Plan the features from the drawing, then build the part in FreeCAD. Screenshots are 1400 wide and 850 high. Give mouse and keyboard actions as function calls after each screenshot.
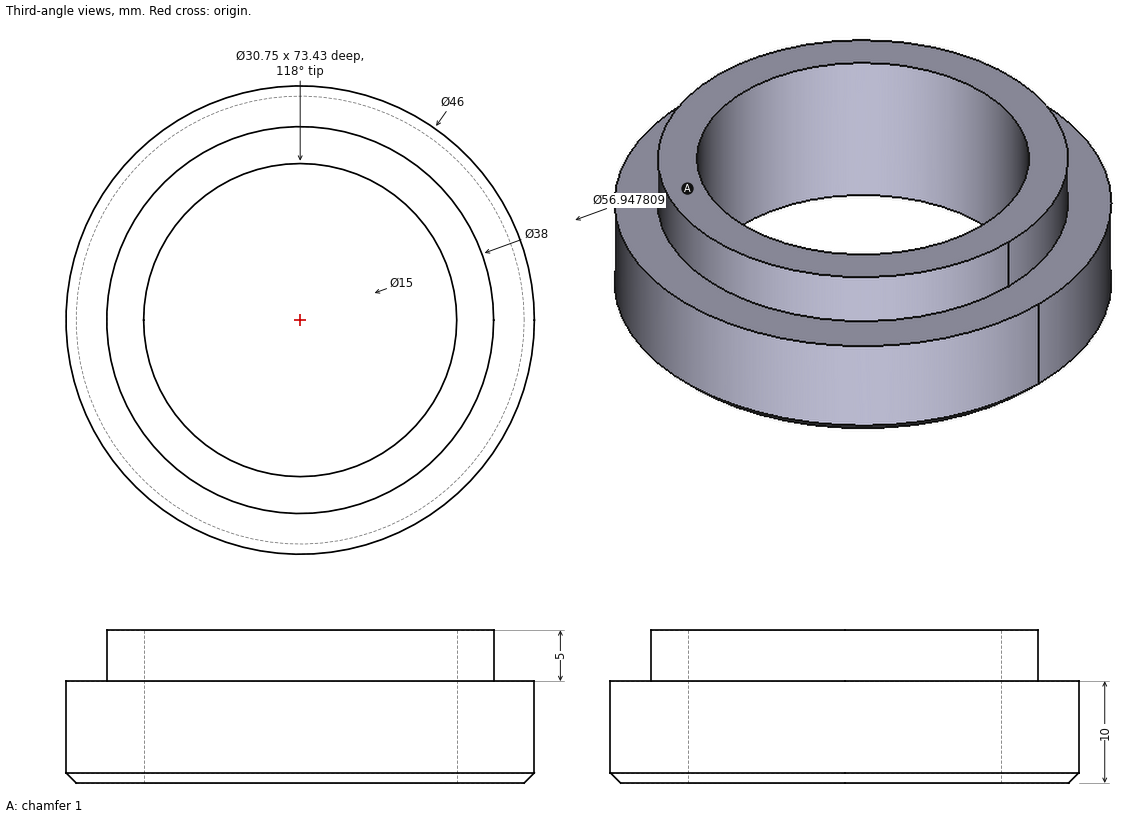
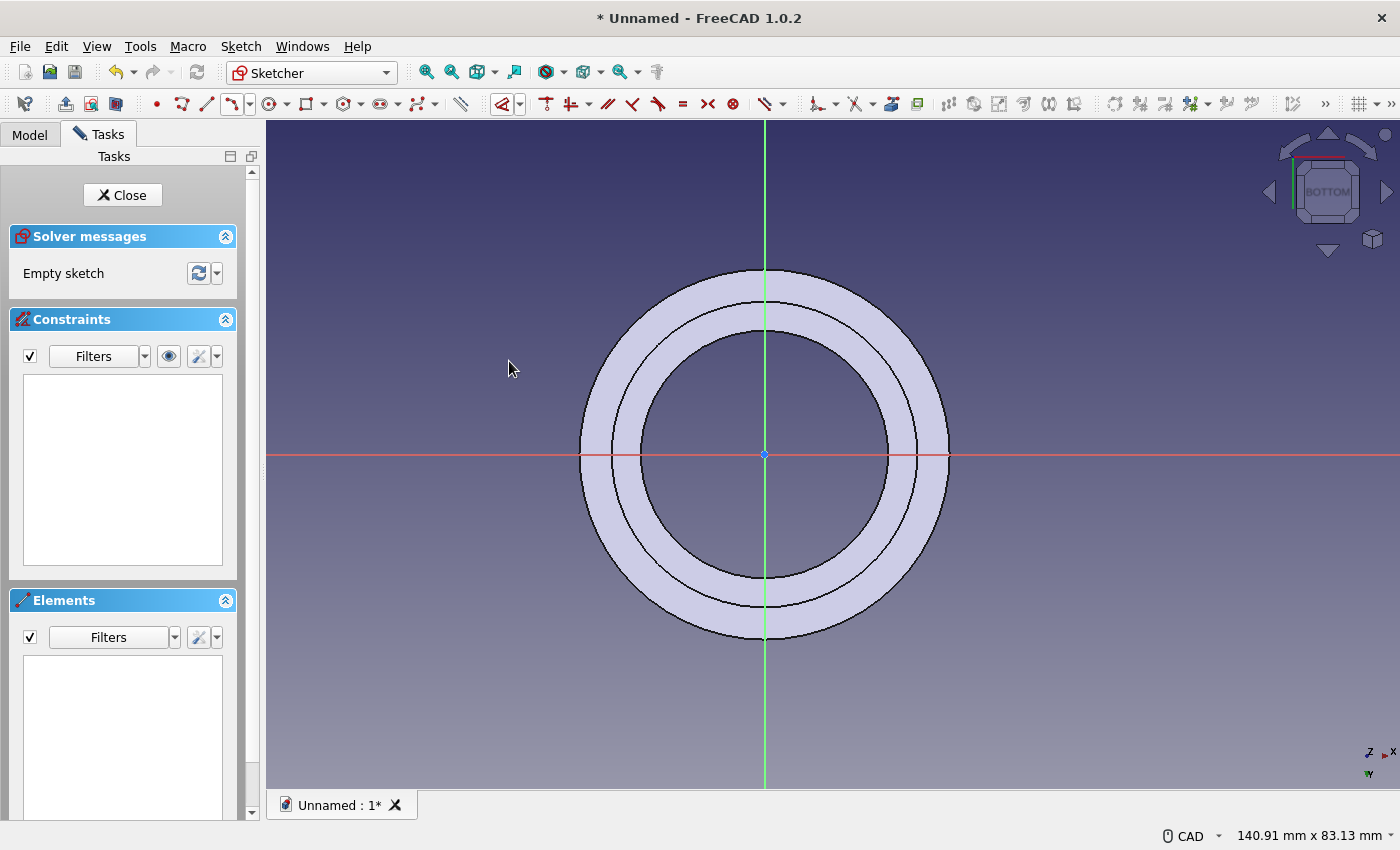
click(268, 104)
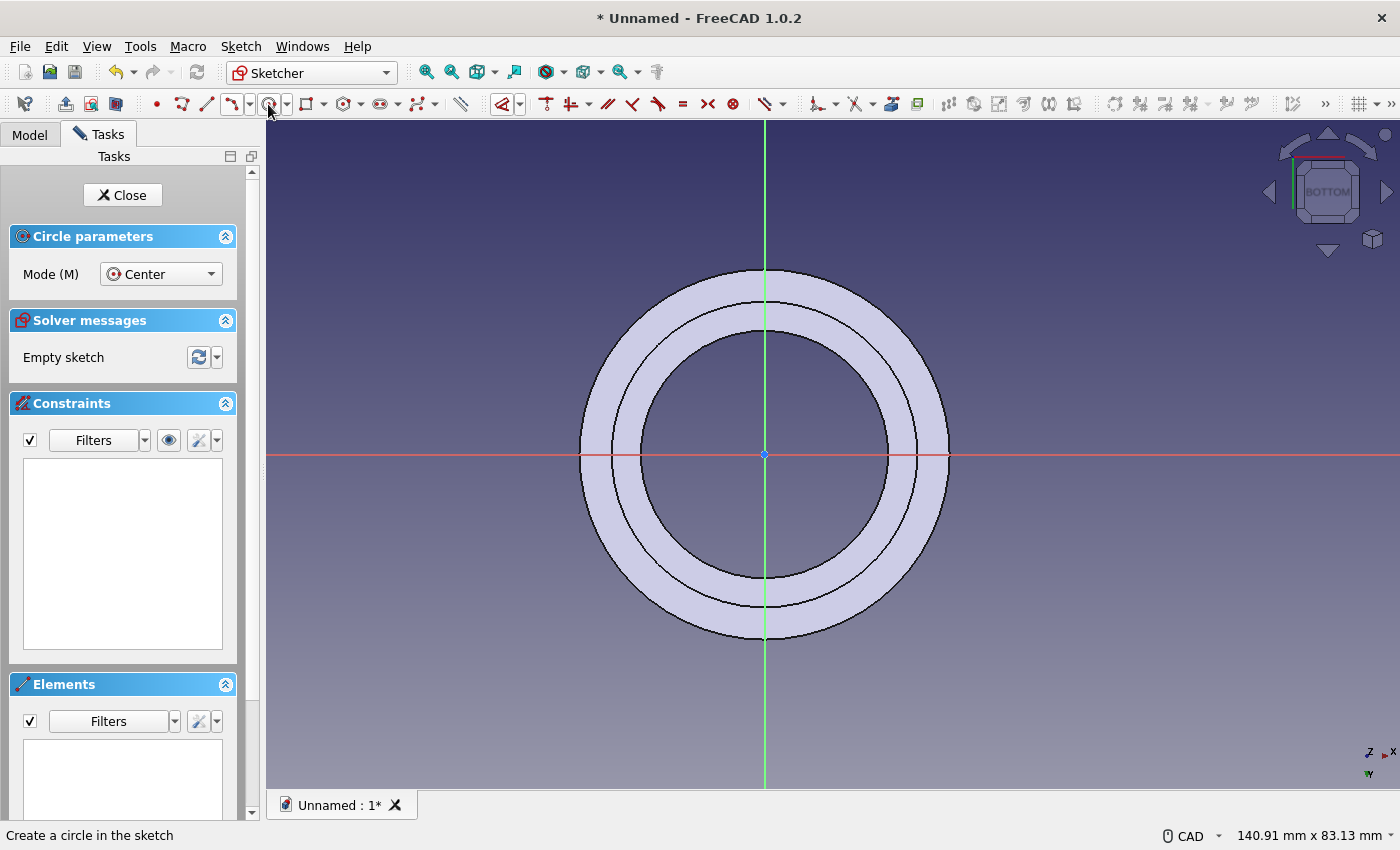
click(765, 455)
move(927, 292)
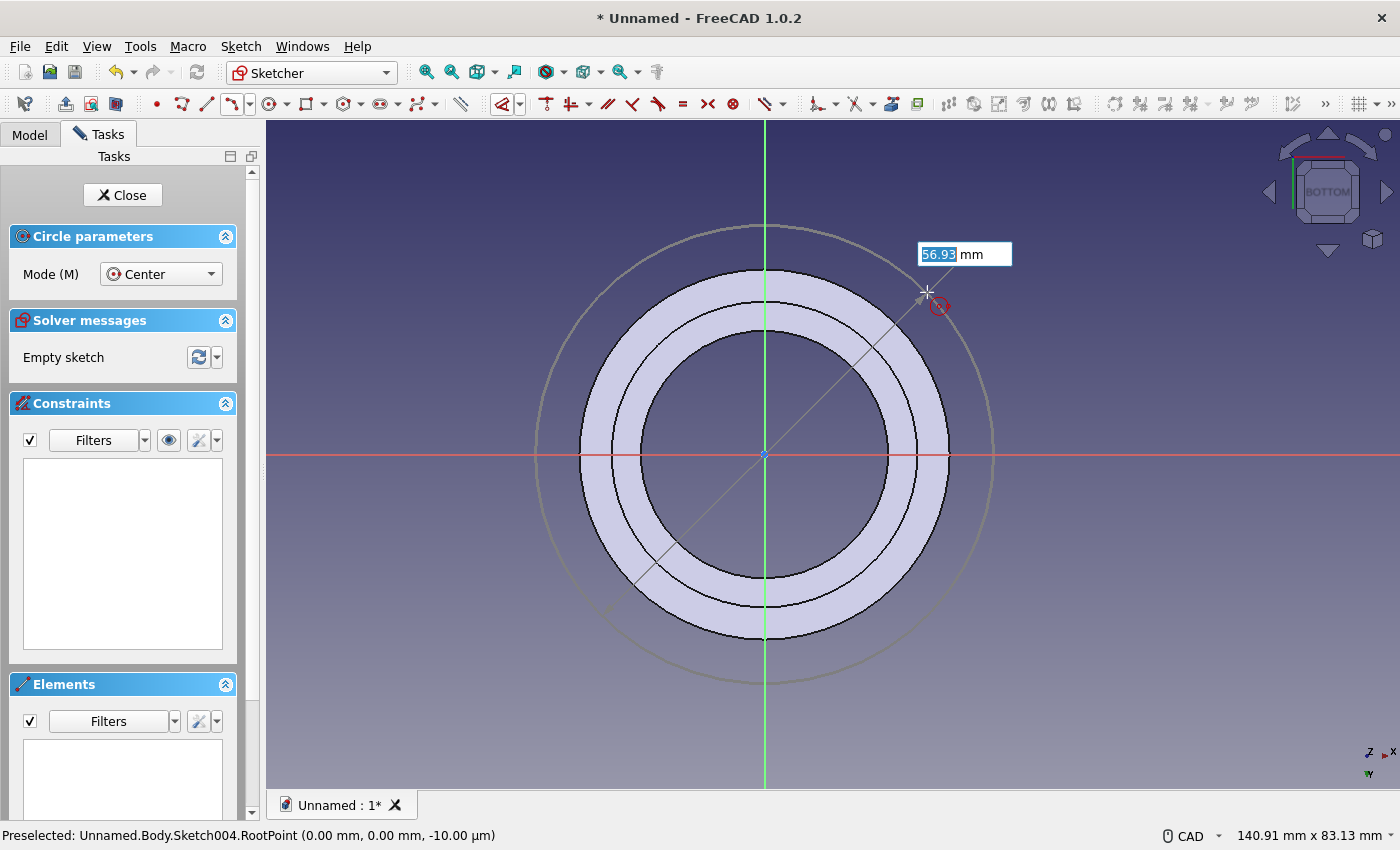
text(56.947809)
key(Return)
key(Escape)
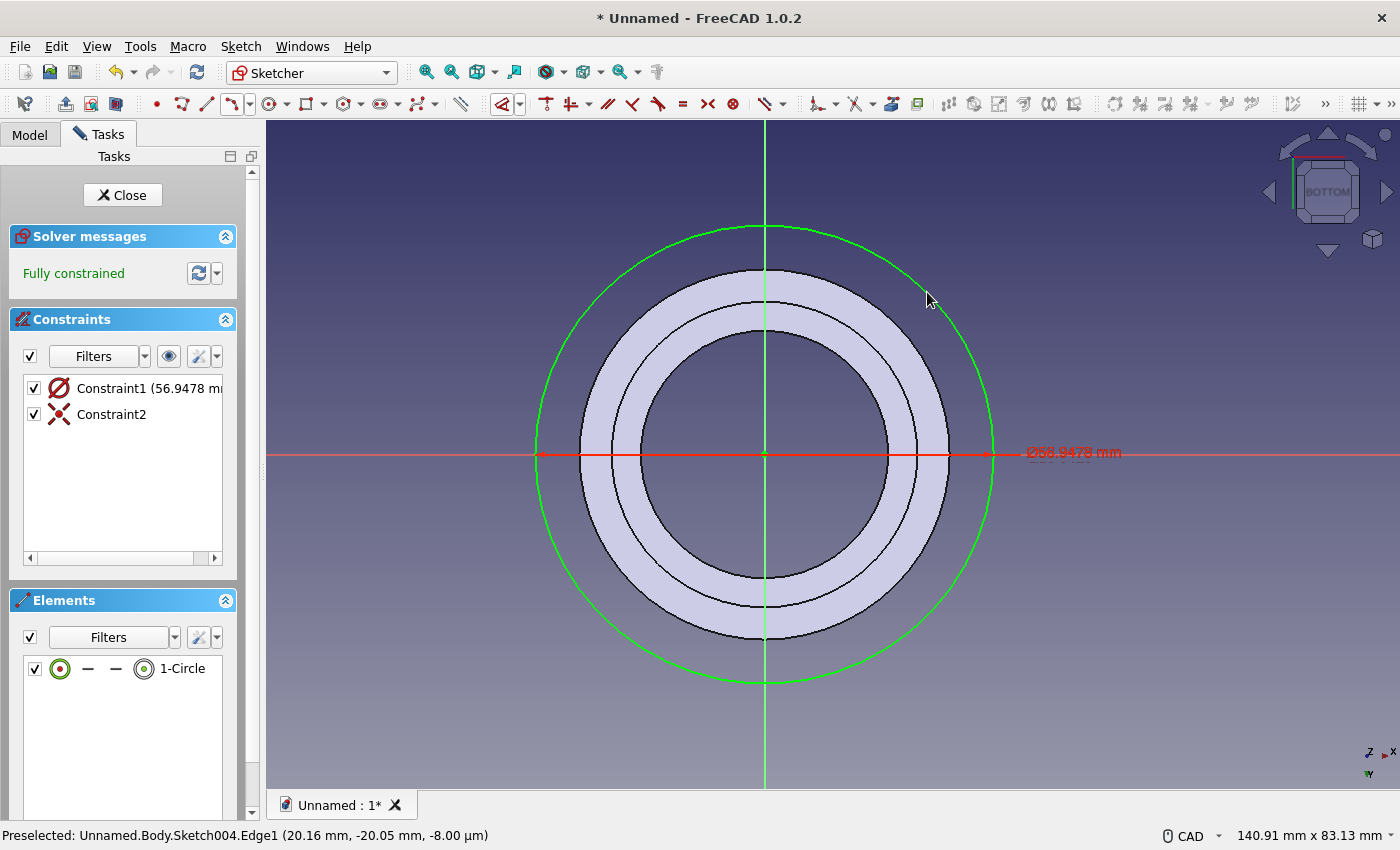
click(123, 195)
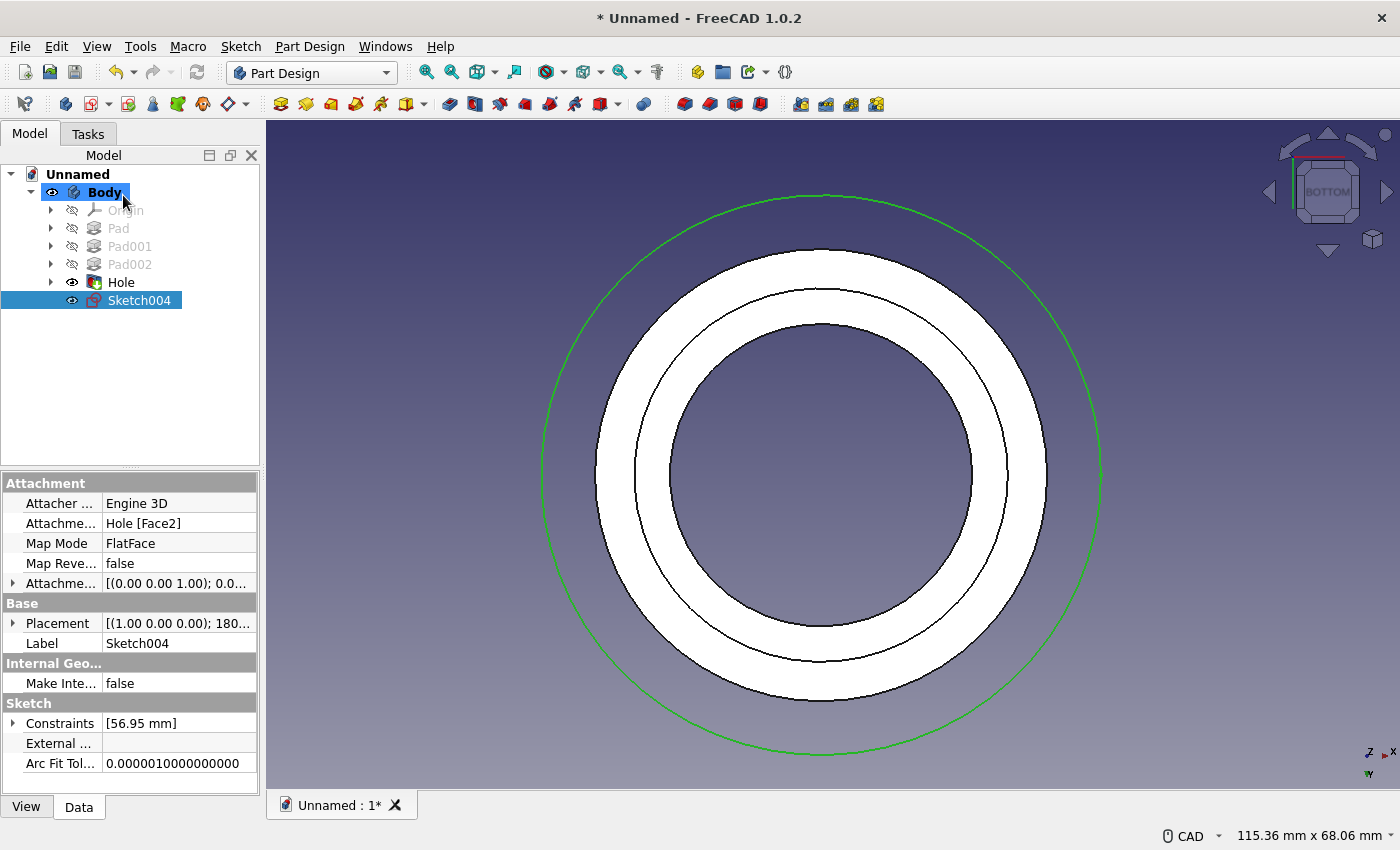
click(450, 104)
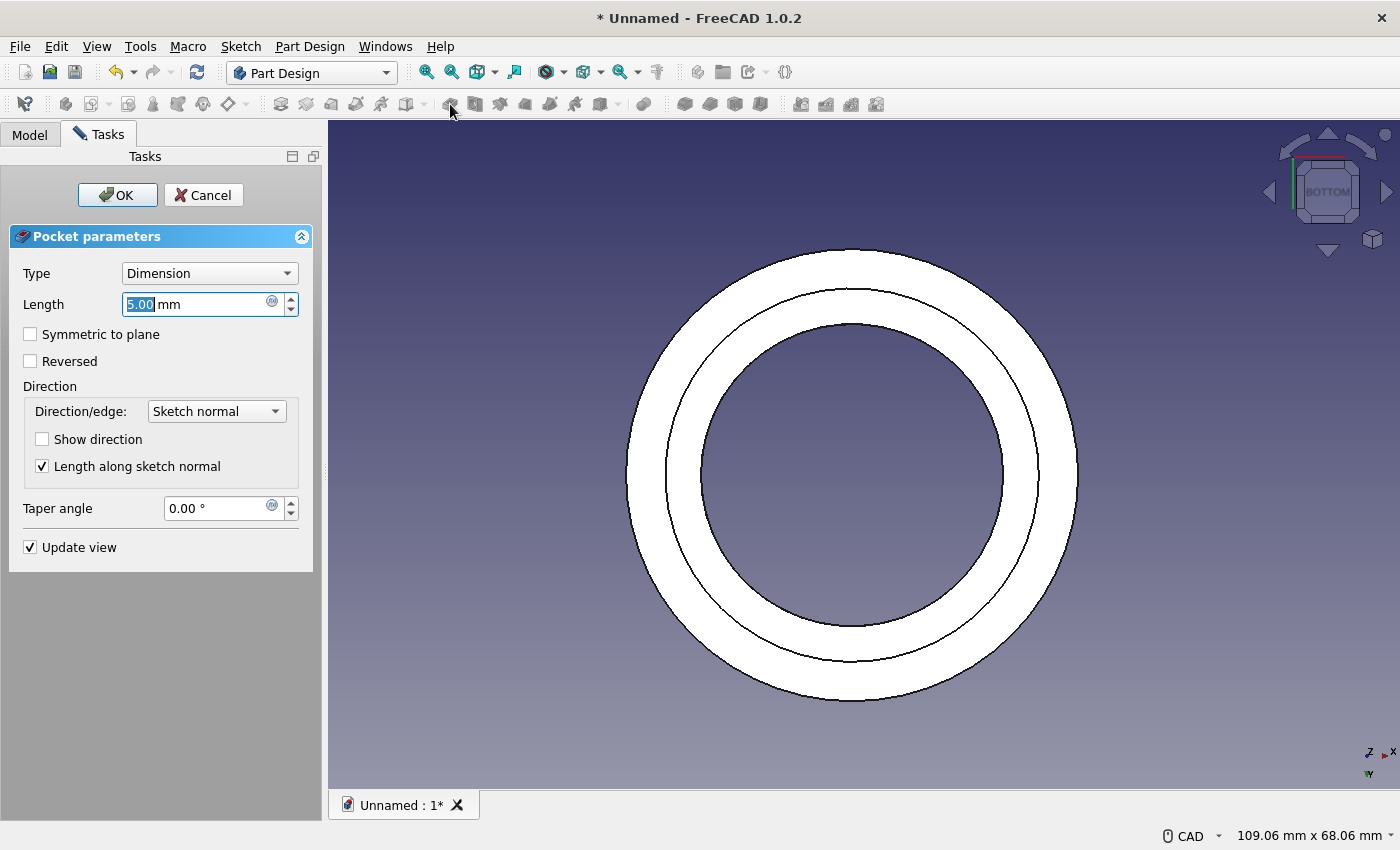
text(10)
key(Tab)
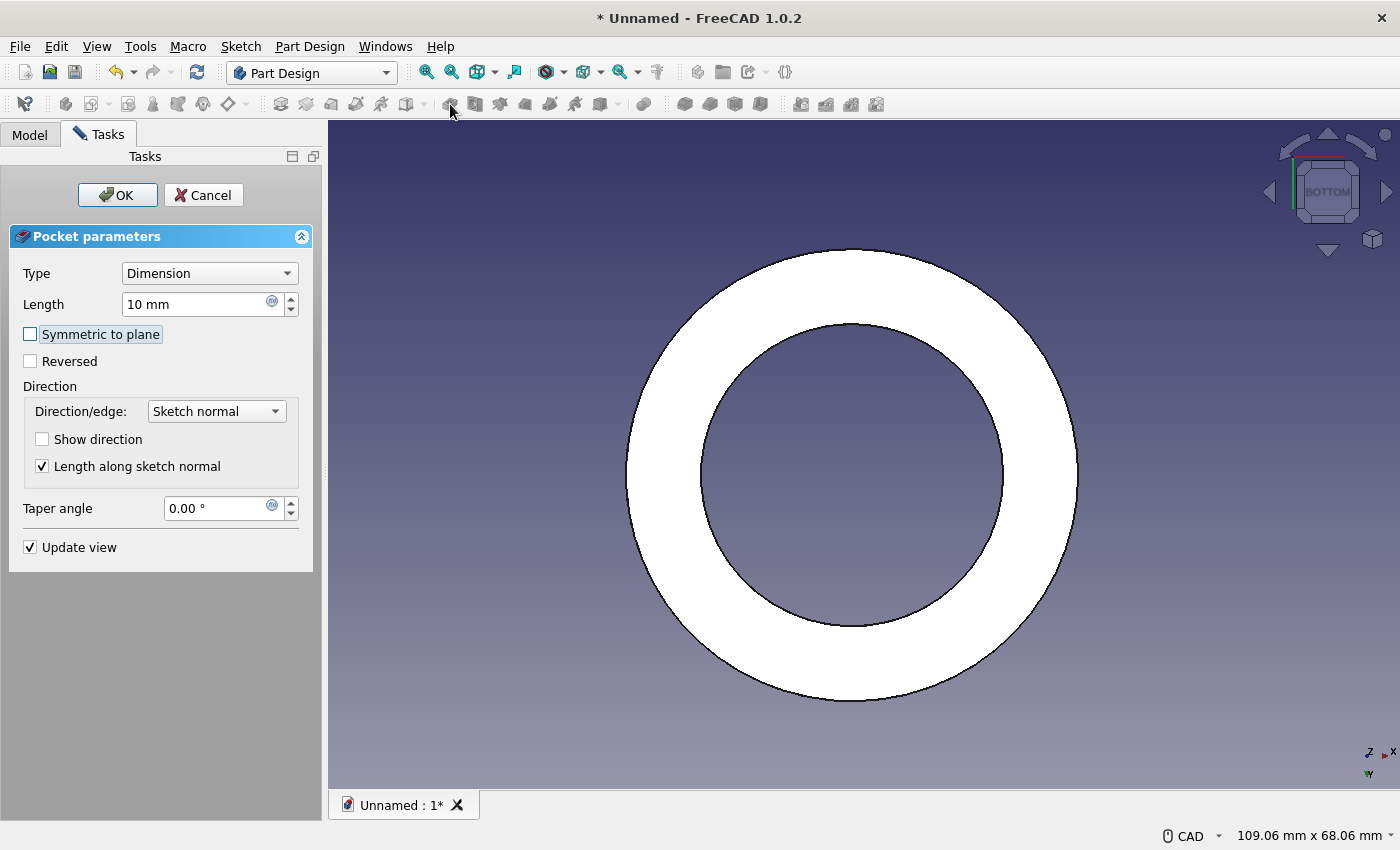
click(118, 195)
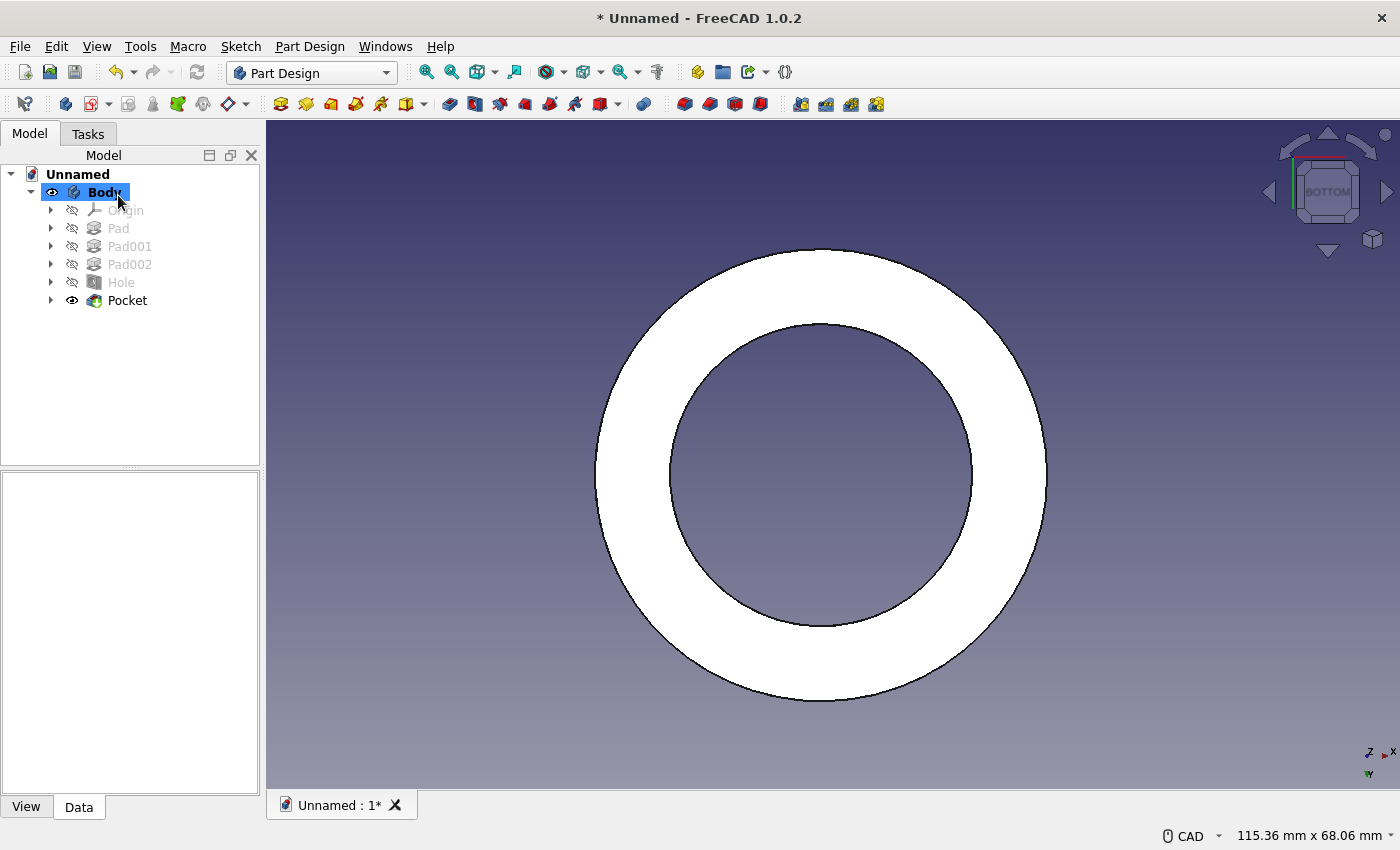
click(595, 474)